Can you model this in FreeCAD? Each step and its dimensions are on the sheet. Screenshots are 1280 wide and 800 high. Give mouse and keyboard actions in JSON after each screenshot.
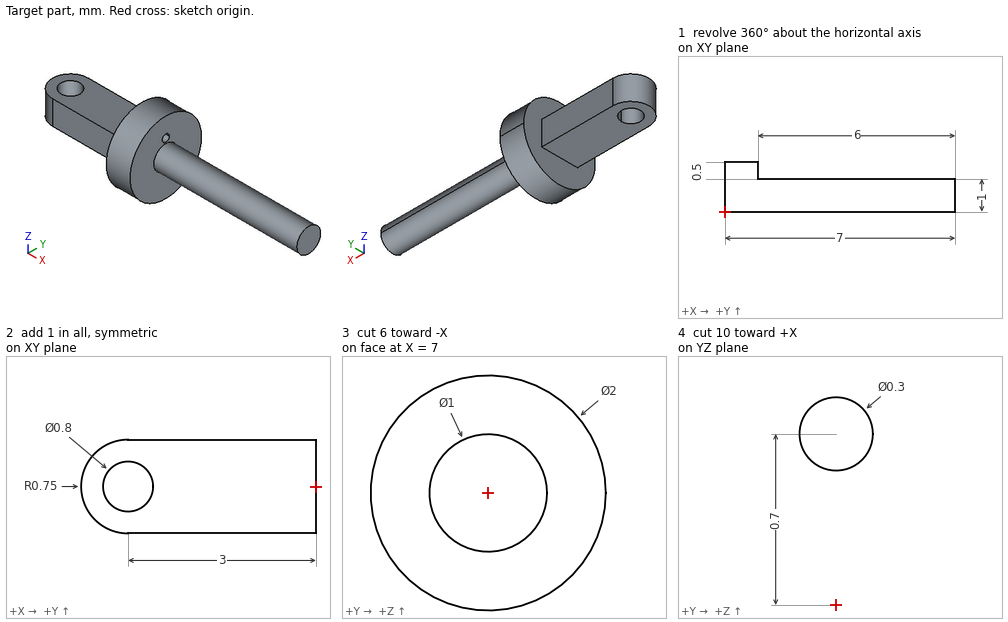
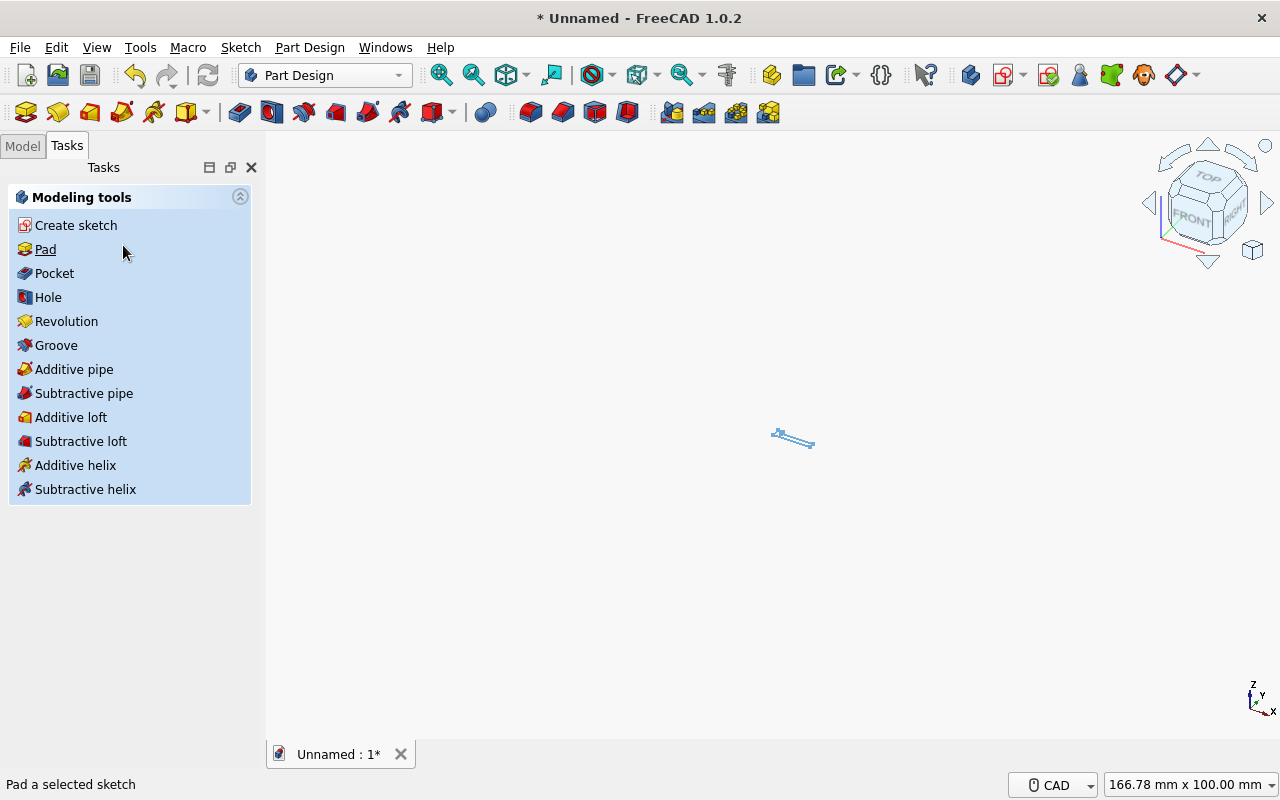
{"action": "left_click", "coordinate": [58, 112]}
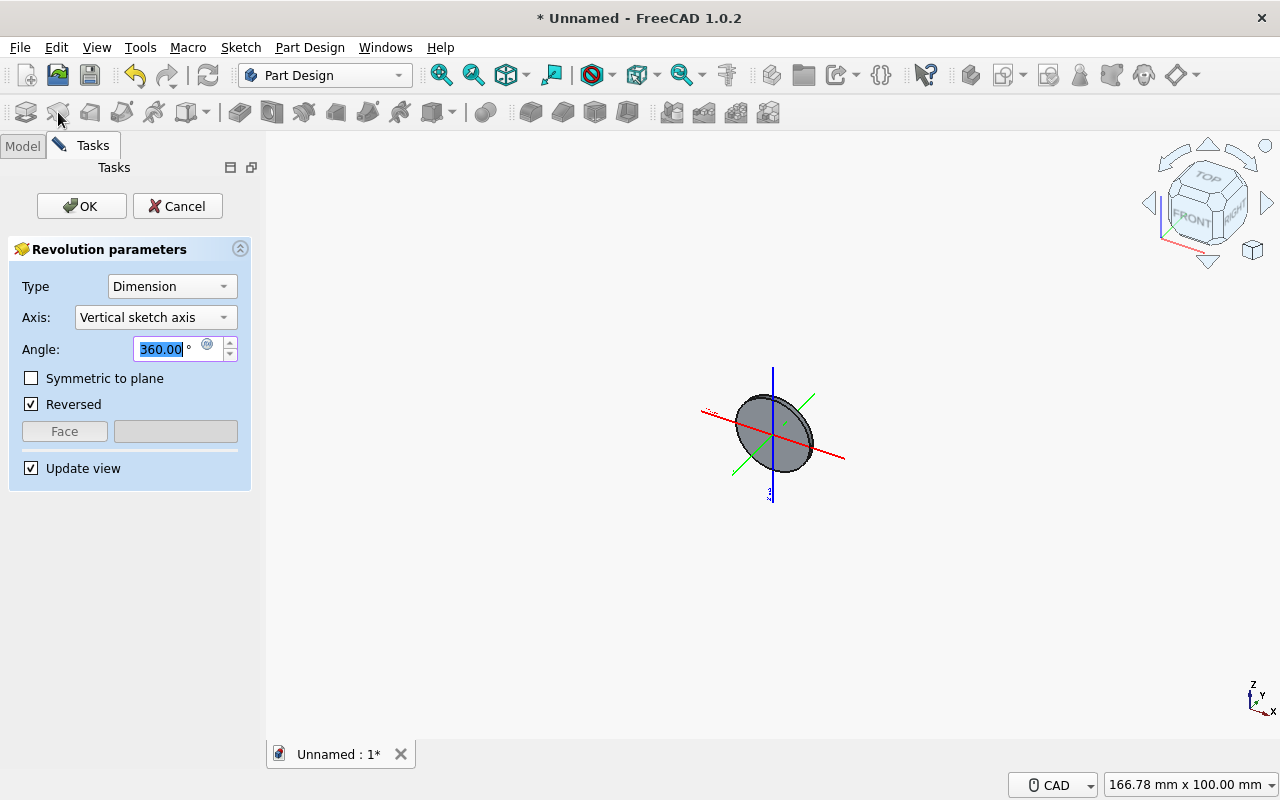
{"action": "left_click", "coordinate": [156, 318]}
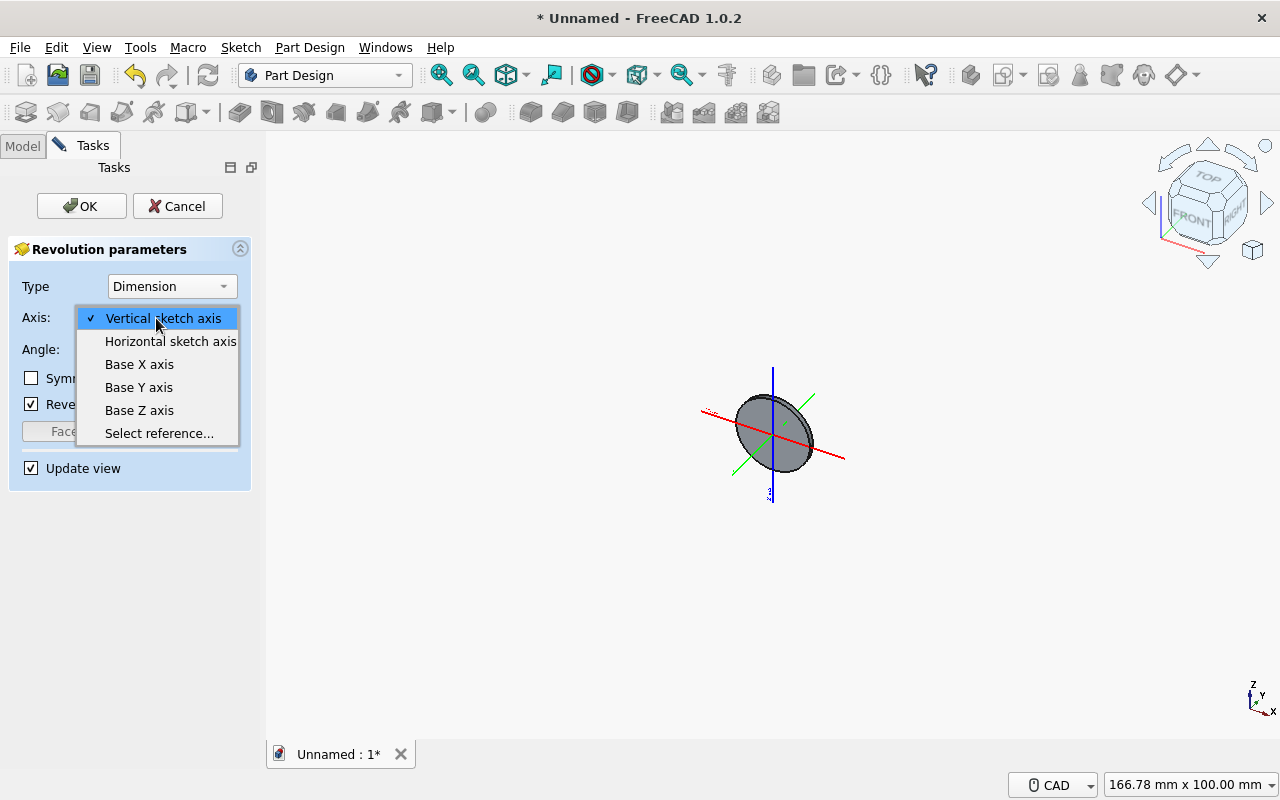
{"action": "left_click", "coordinate": [156, 342]}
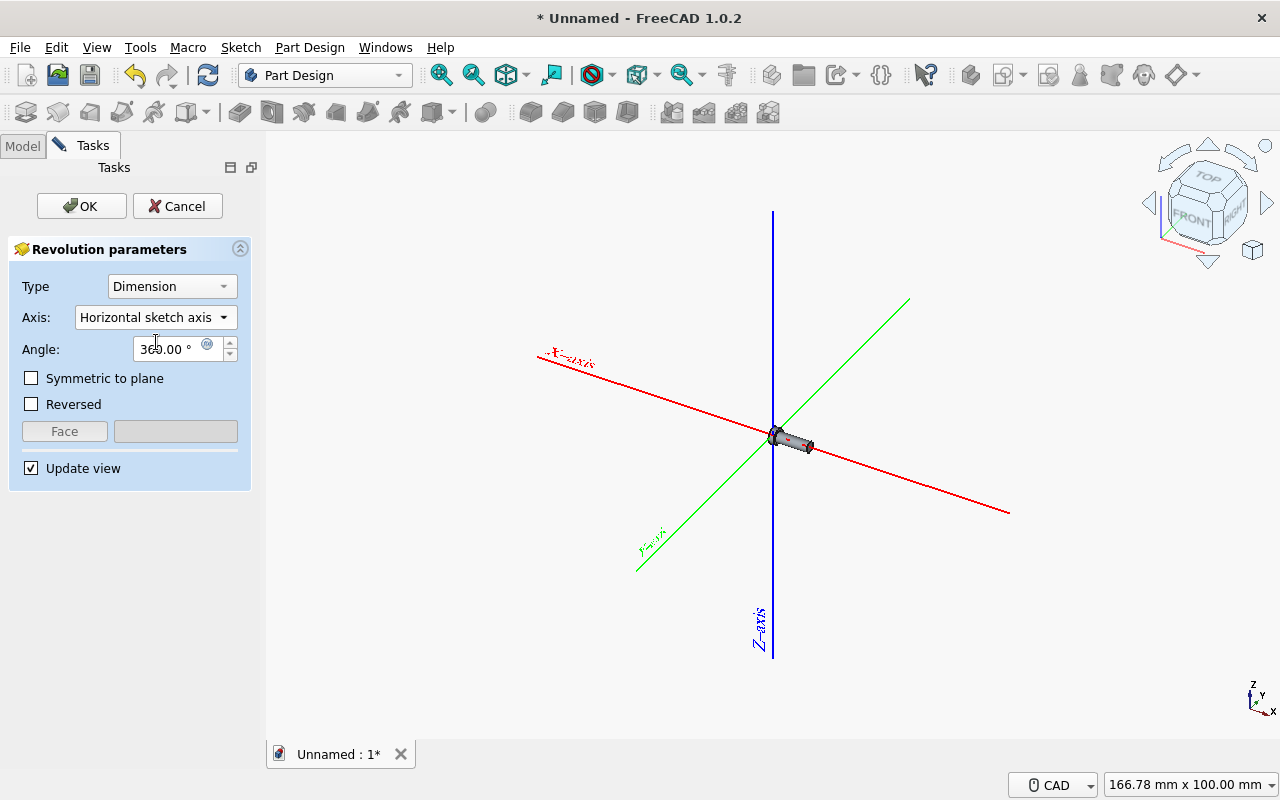
{"action": "left_click", "coordinate": [82, 206]}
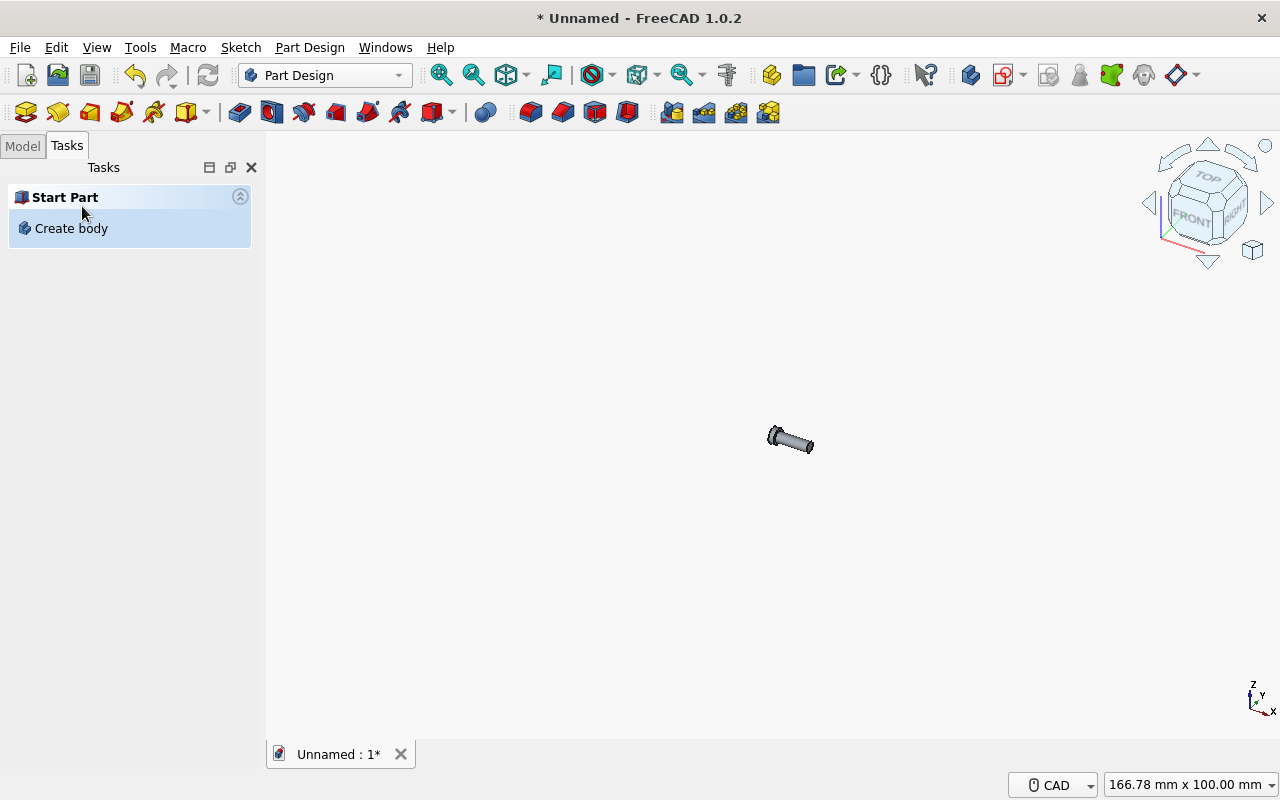
{"action": "left_click", "coordinate": [442, 76]}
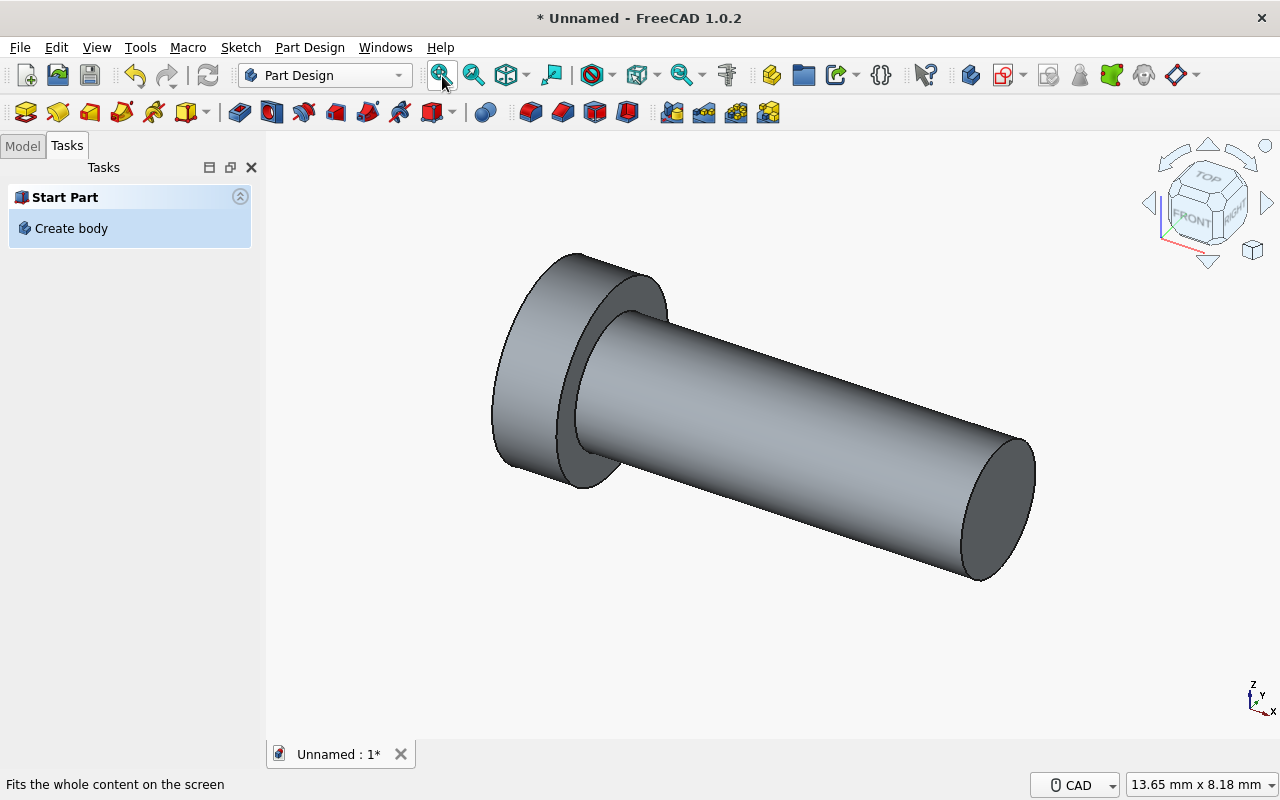
{"action": "left_click", "coordinate": [1004, 76]}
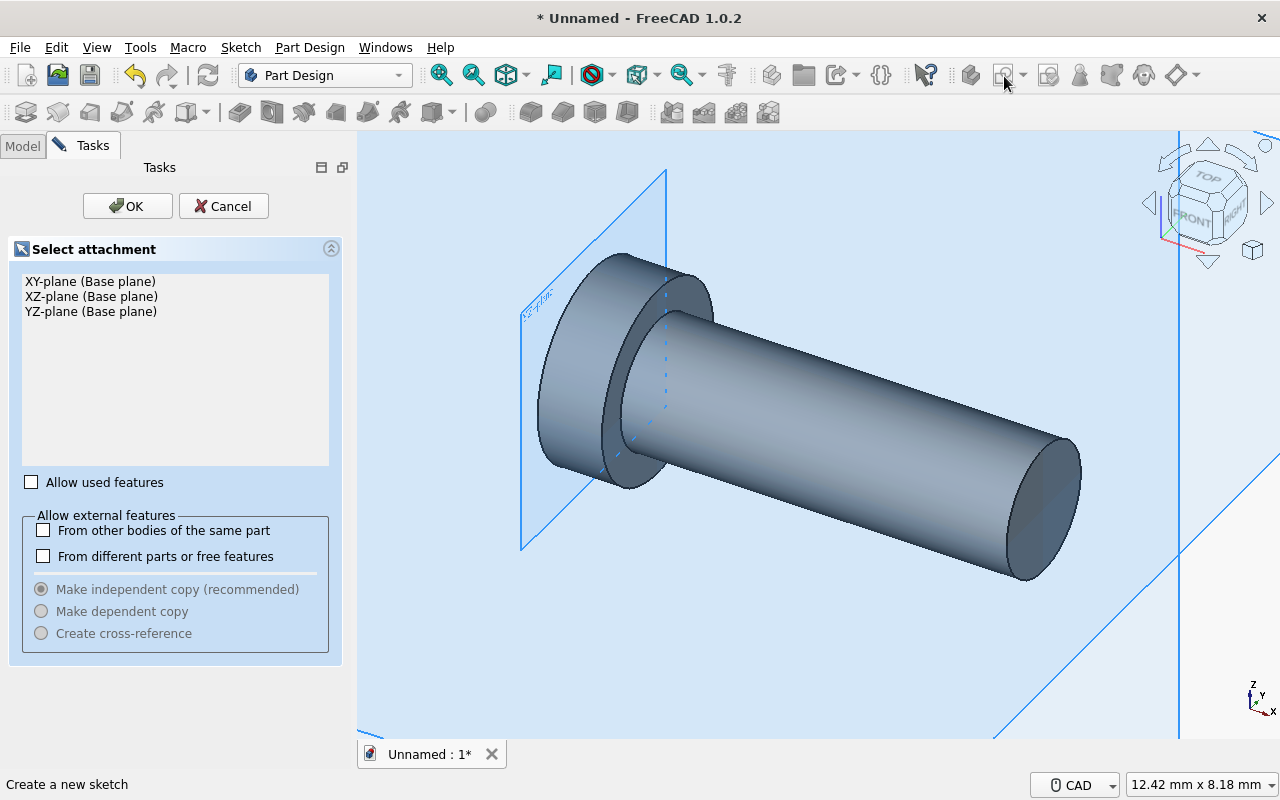
{"action": "left_click", "coordinate": [82, 282]}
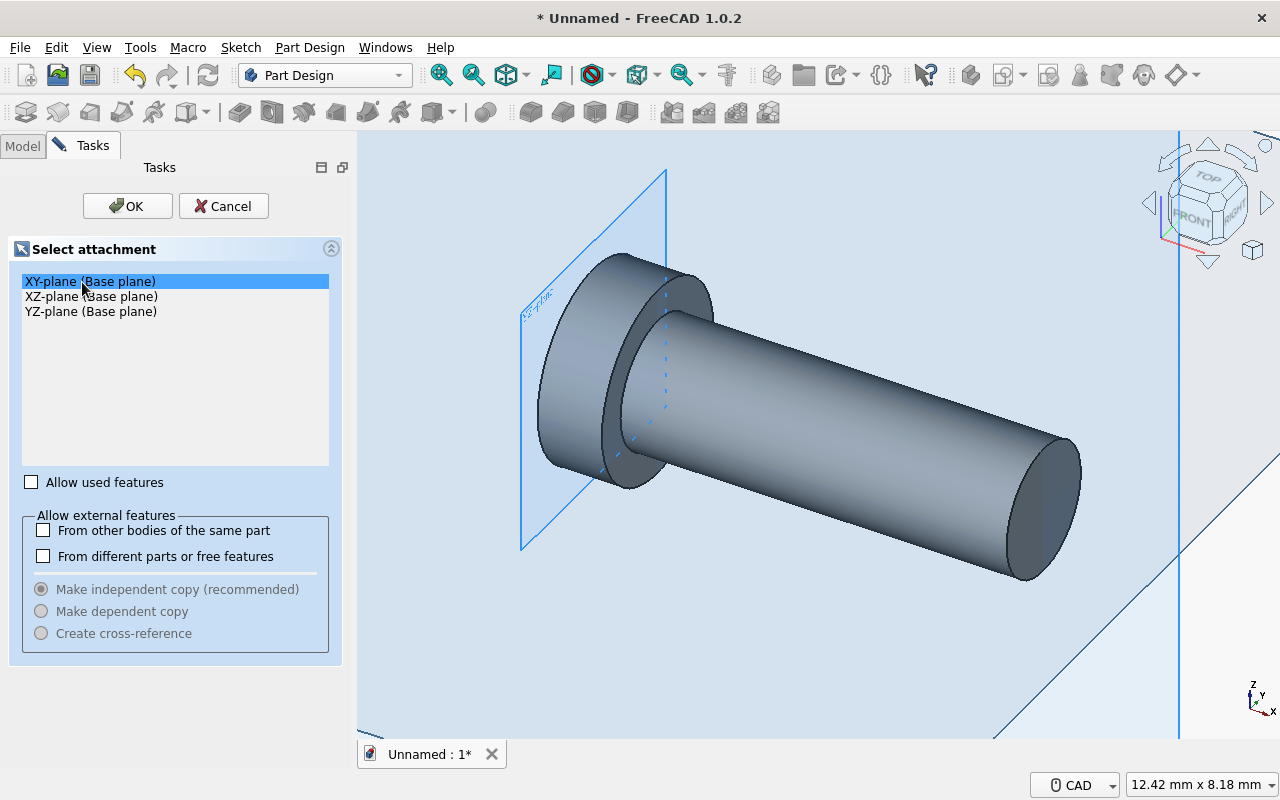
{"action": "left_click", "coordinate": [128, 206]}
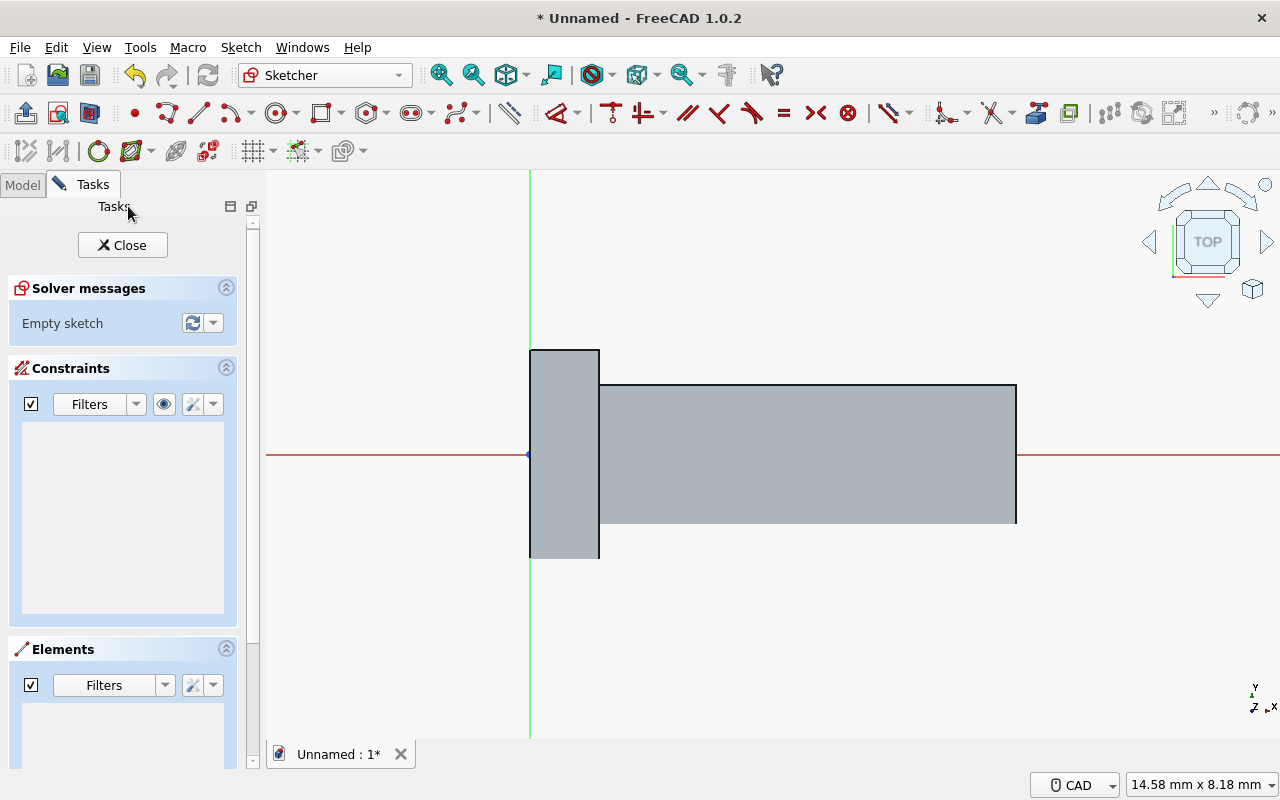
{"action": "left_click", "coordinate": [90, 114]}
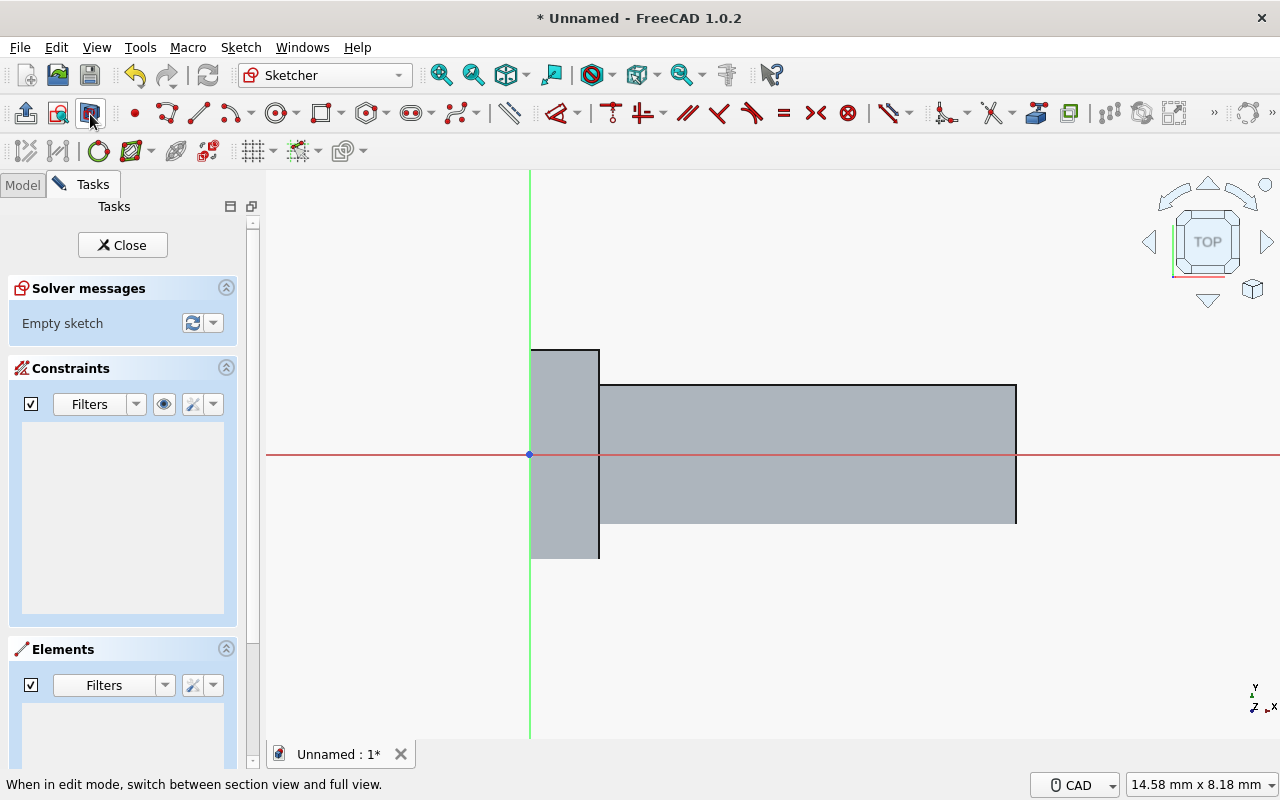
{"action": "scroll", "coordinate": [704, 454], "scroll_direction": "down", "scroll_amount": 5}